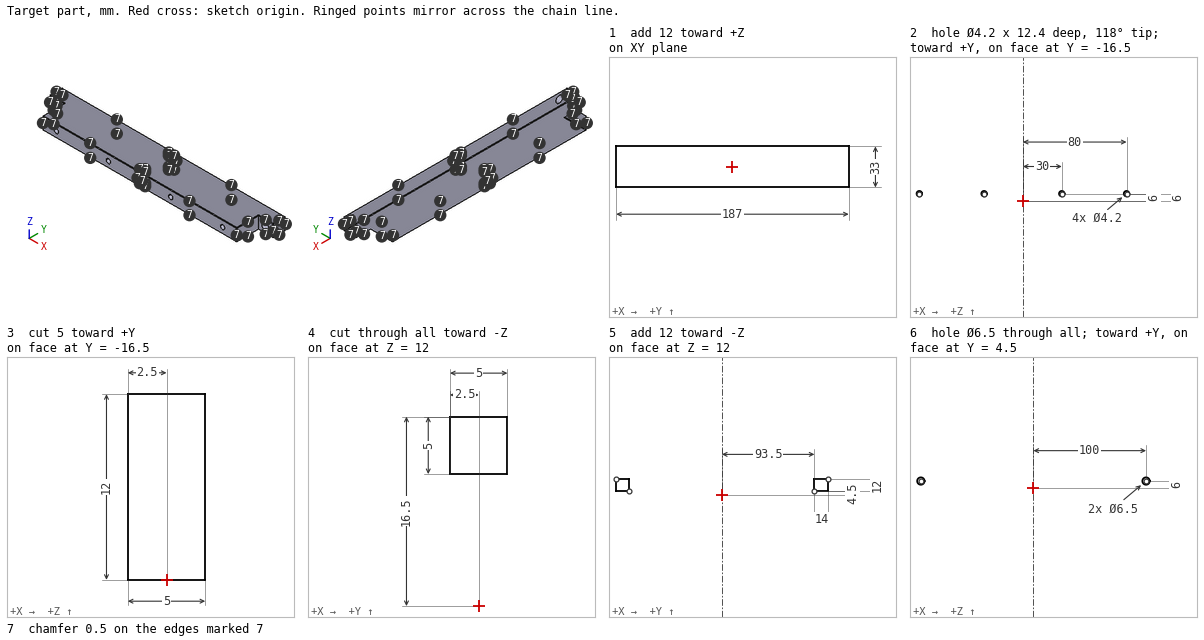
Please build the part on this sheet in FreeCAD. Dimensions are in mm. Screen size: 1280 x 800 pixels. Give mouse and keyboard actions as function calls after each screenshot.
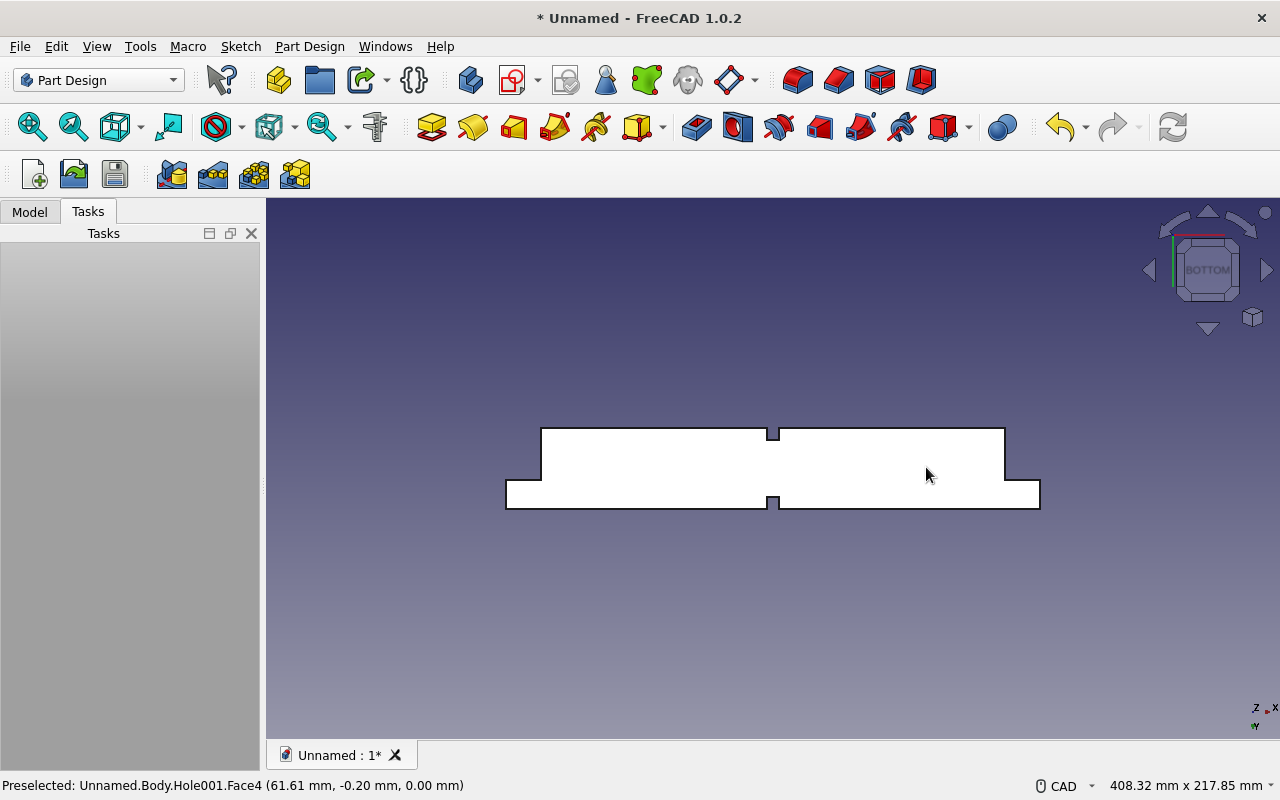
key(4)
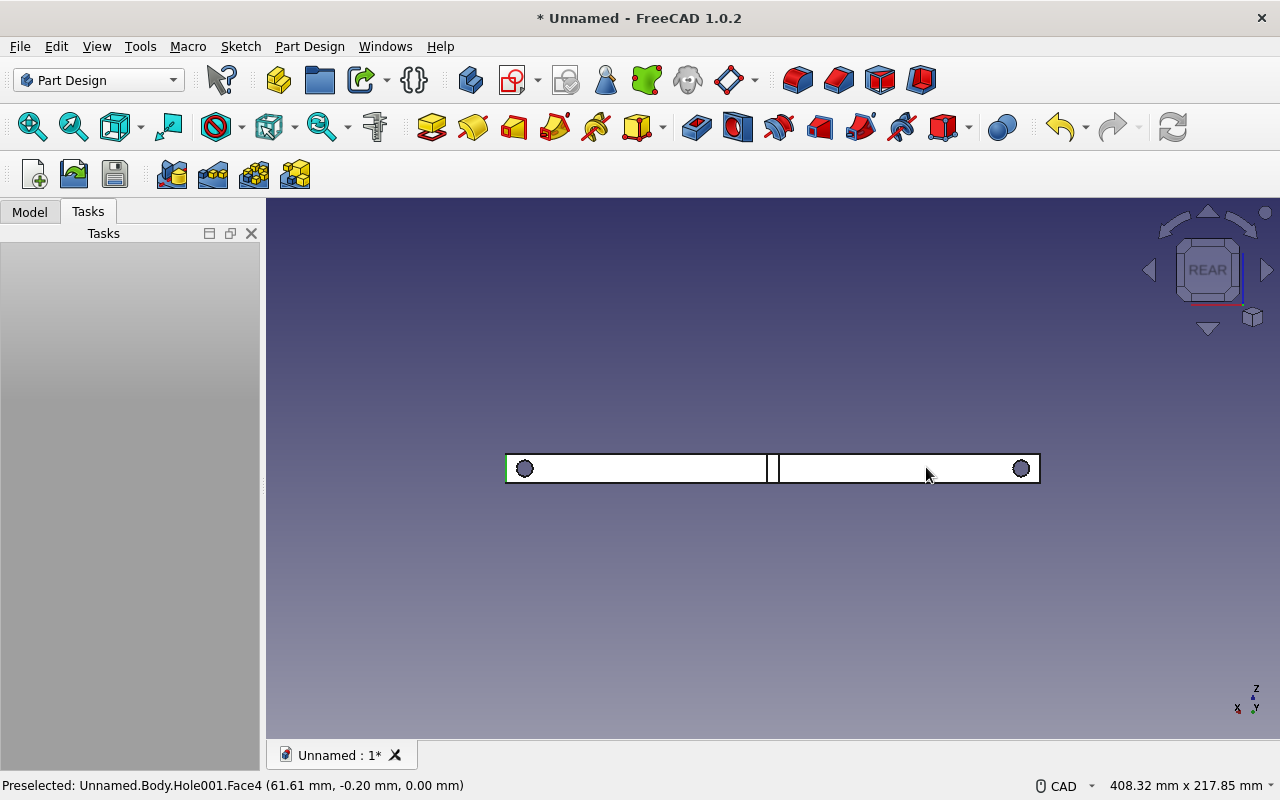
click(779, 467, ctrl)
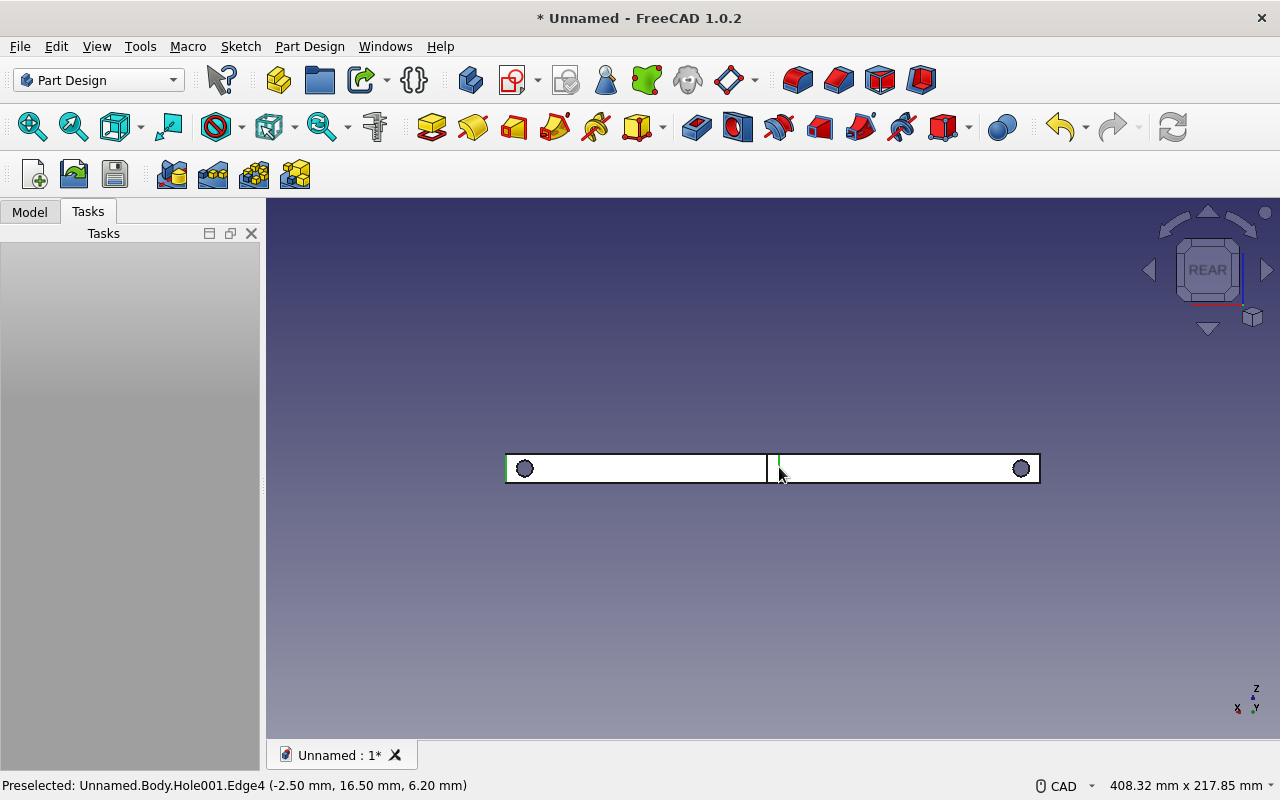
click(767, 467, ctrl)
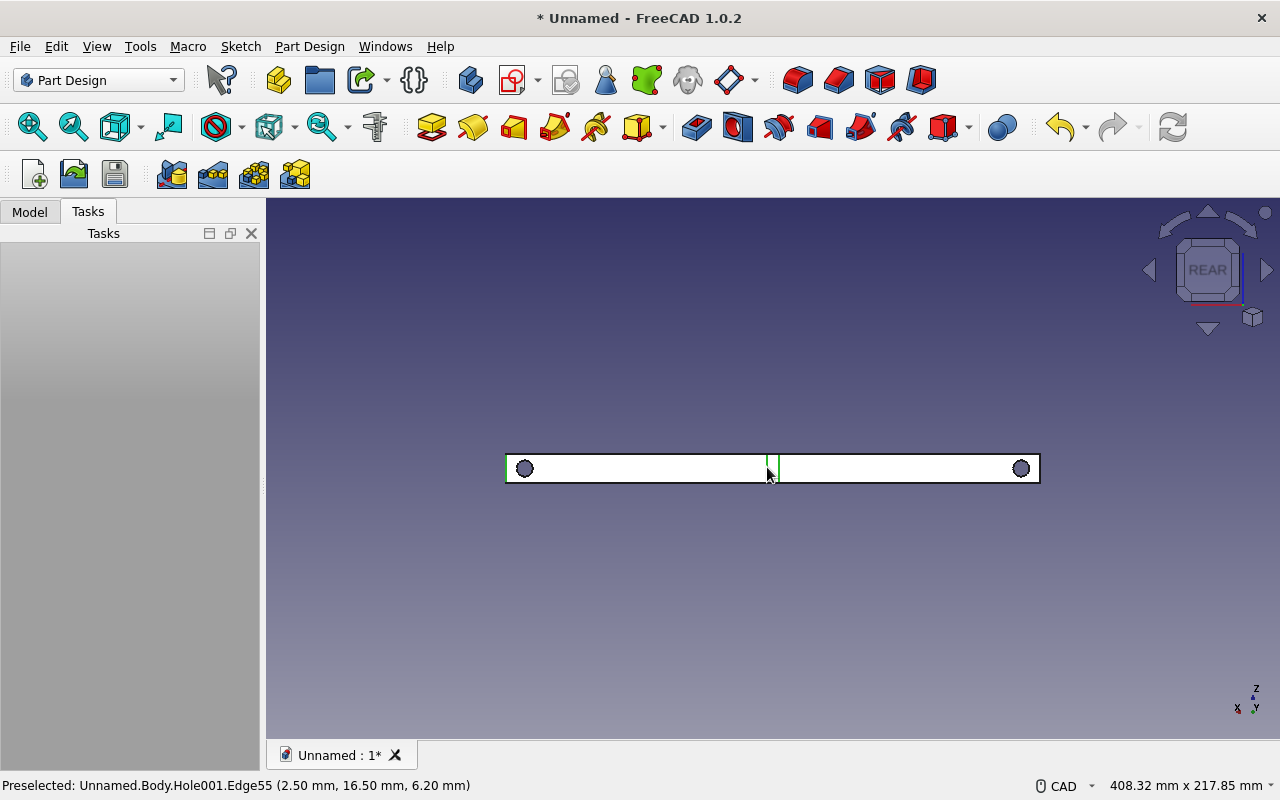
click(1040, 467, ctrl)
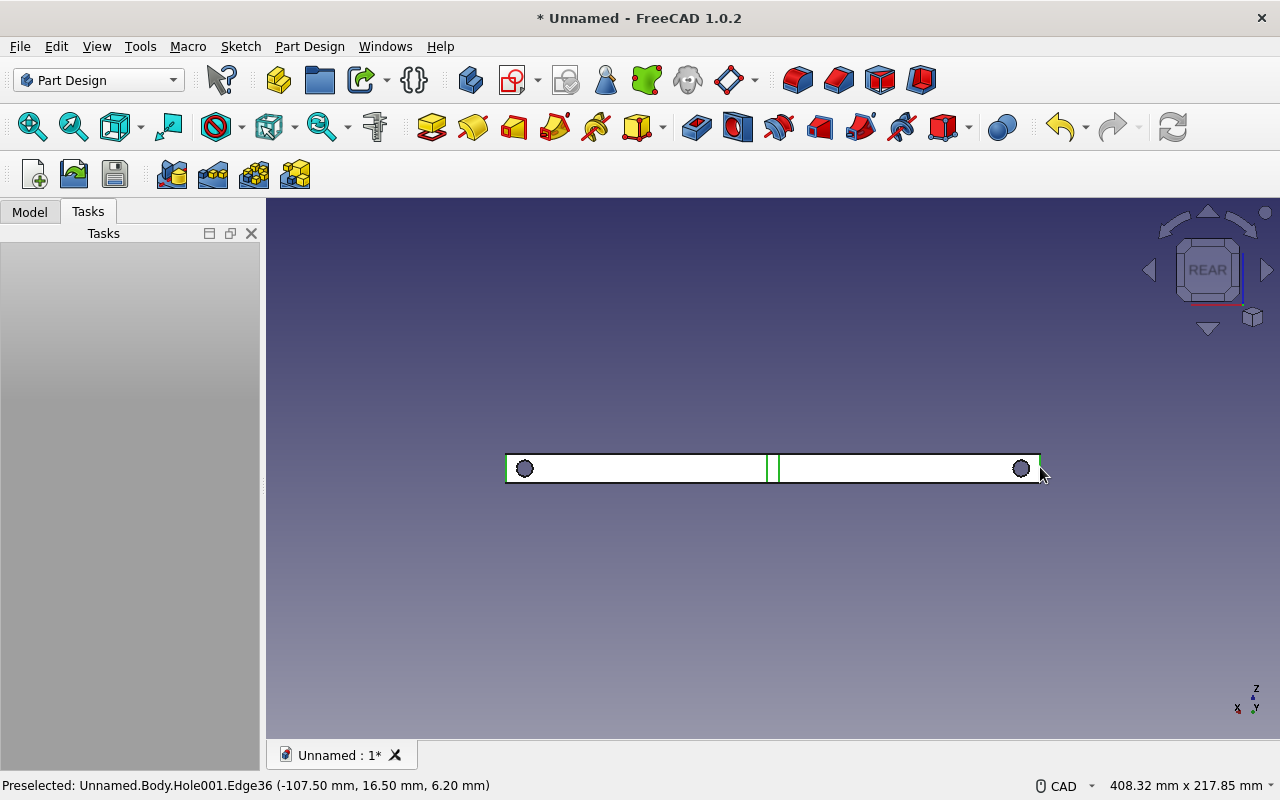
click(839, 80)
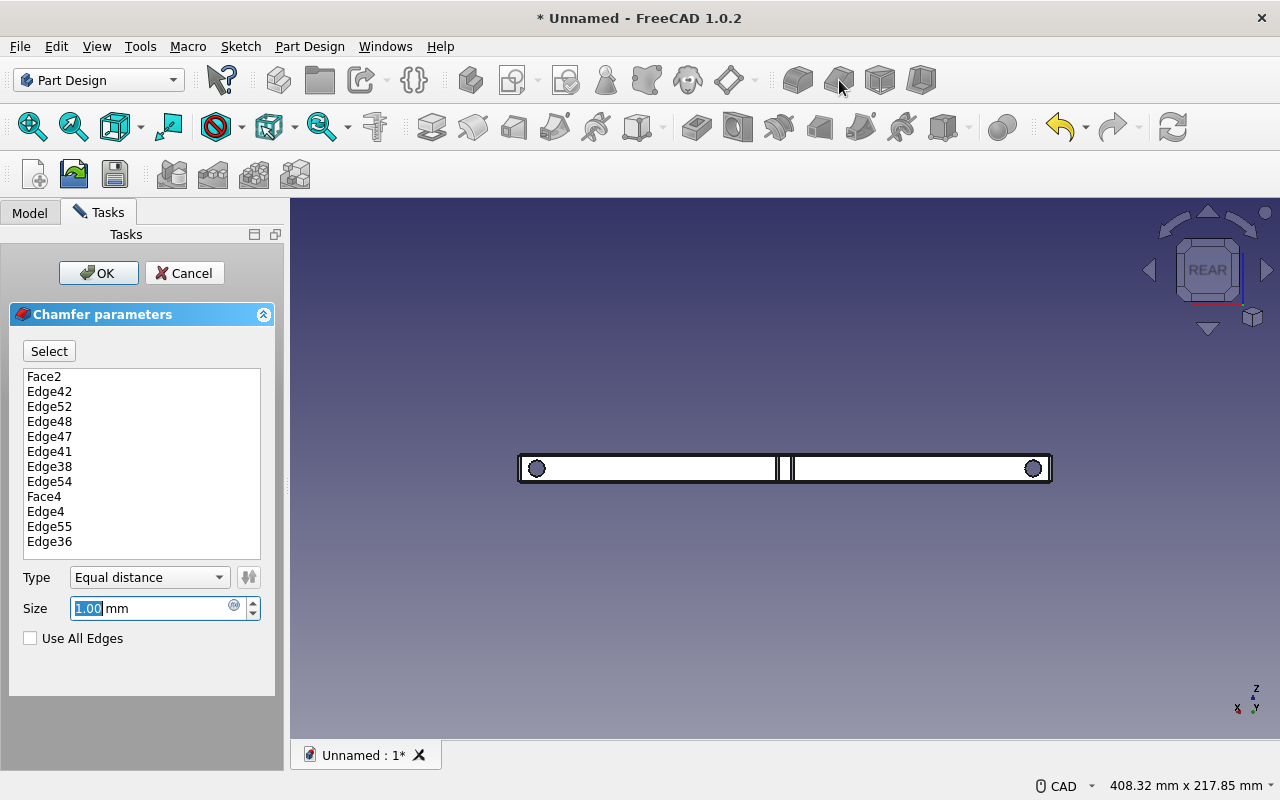
text(0.5)
key(Tab)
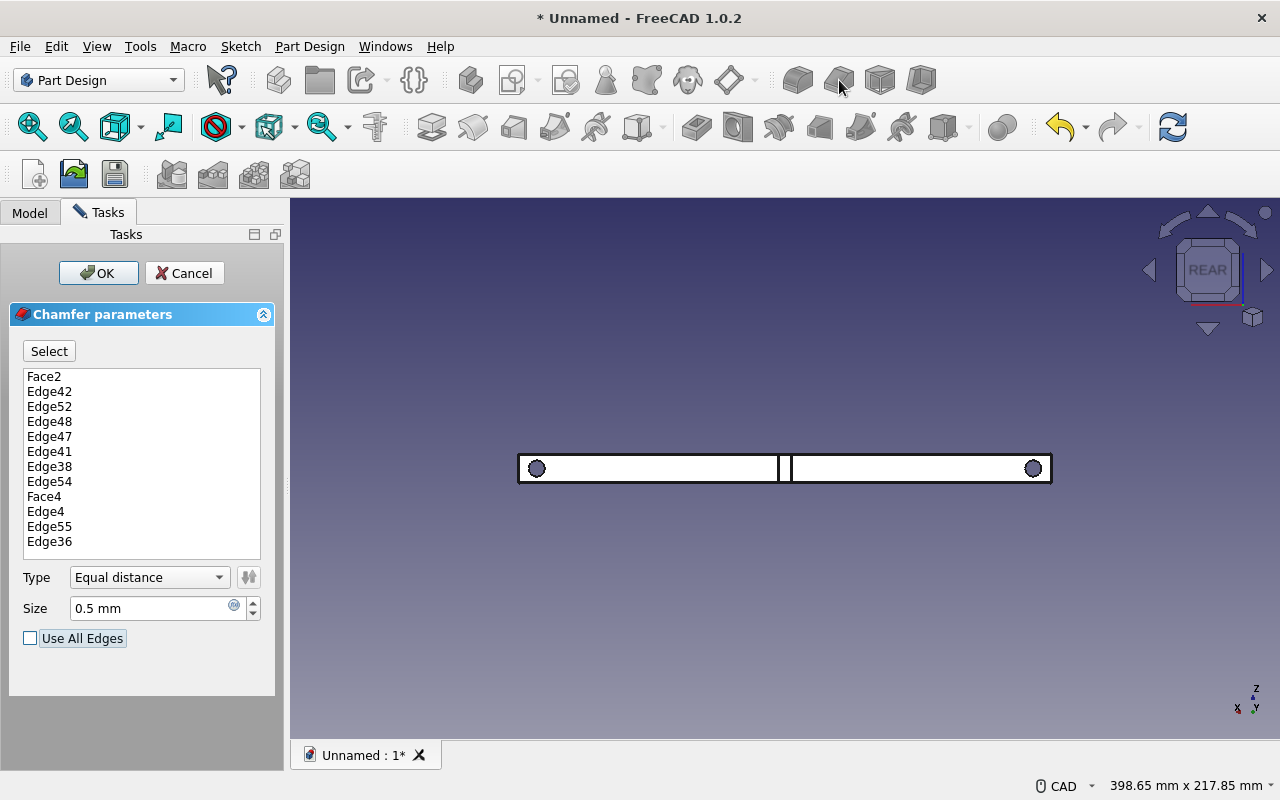
click(99, 273)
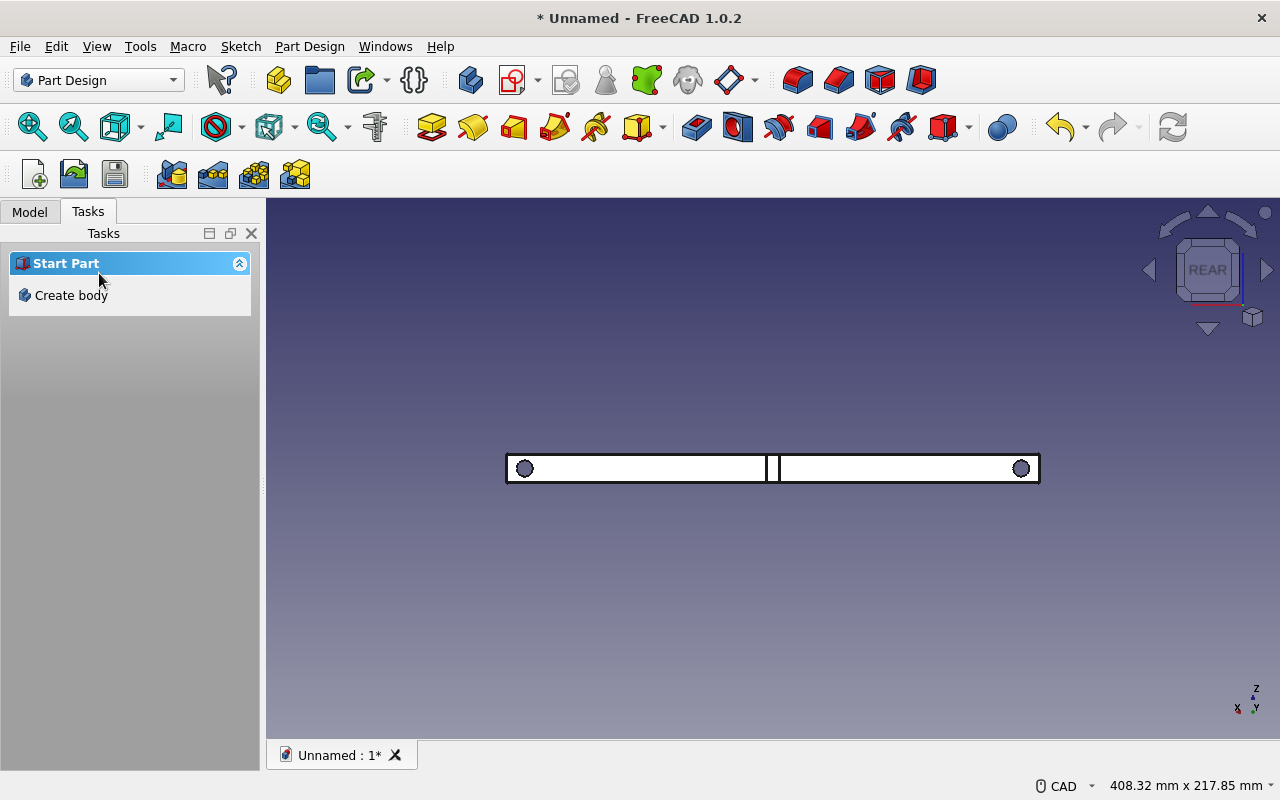
key(0)